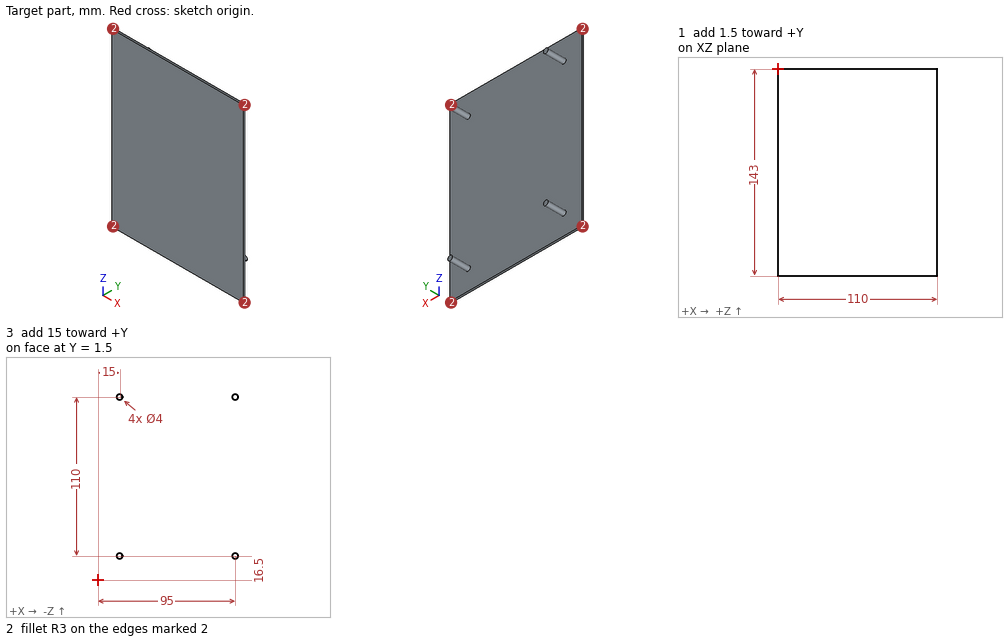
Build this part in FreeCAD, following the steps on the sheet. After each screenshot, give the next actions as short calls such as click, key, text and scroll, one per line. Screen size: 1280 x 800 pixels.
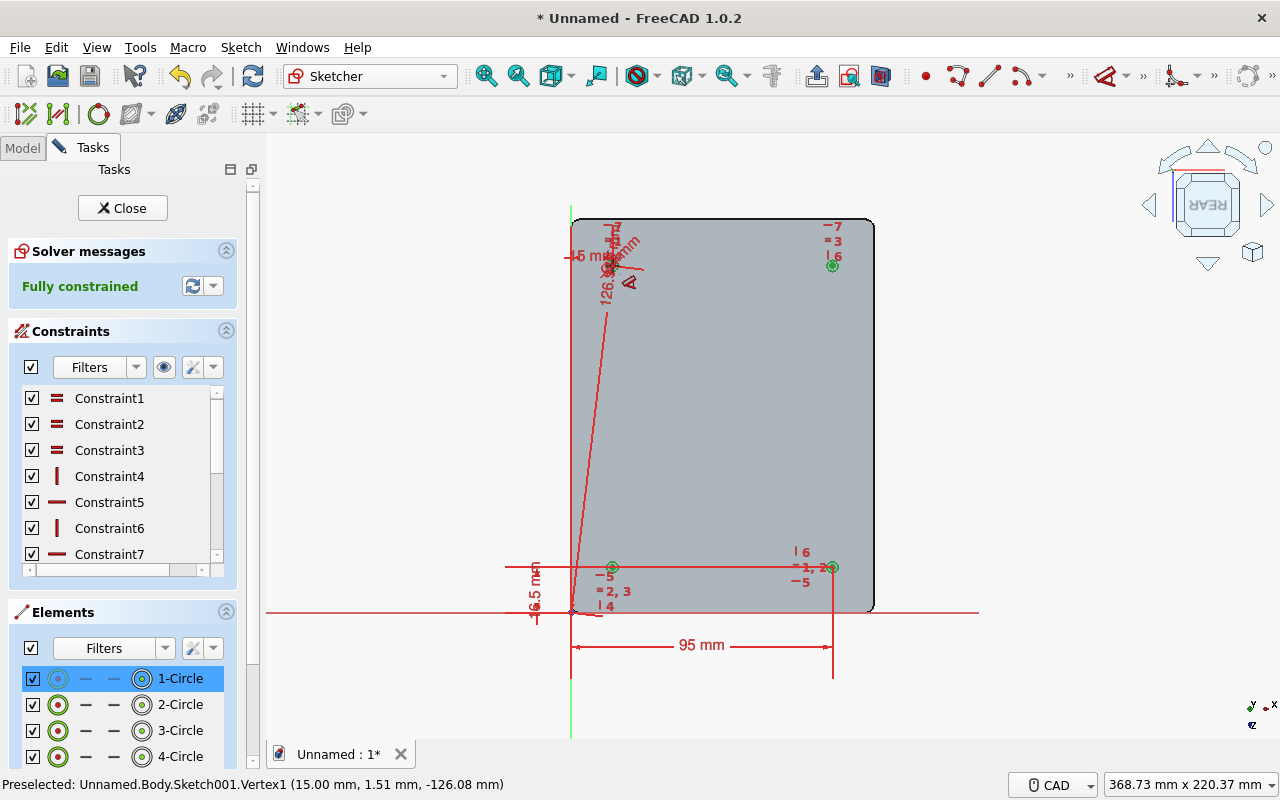
click(833, 567)
click(867, 417)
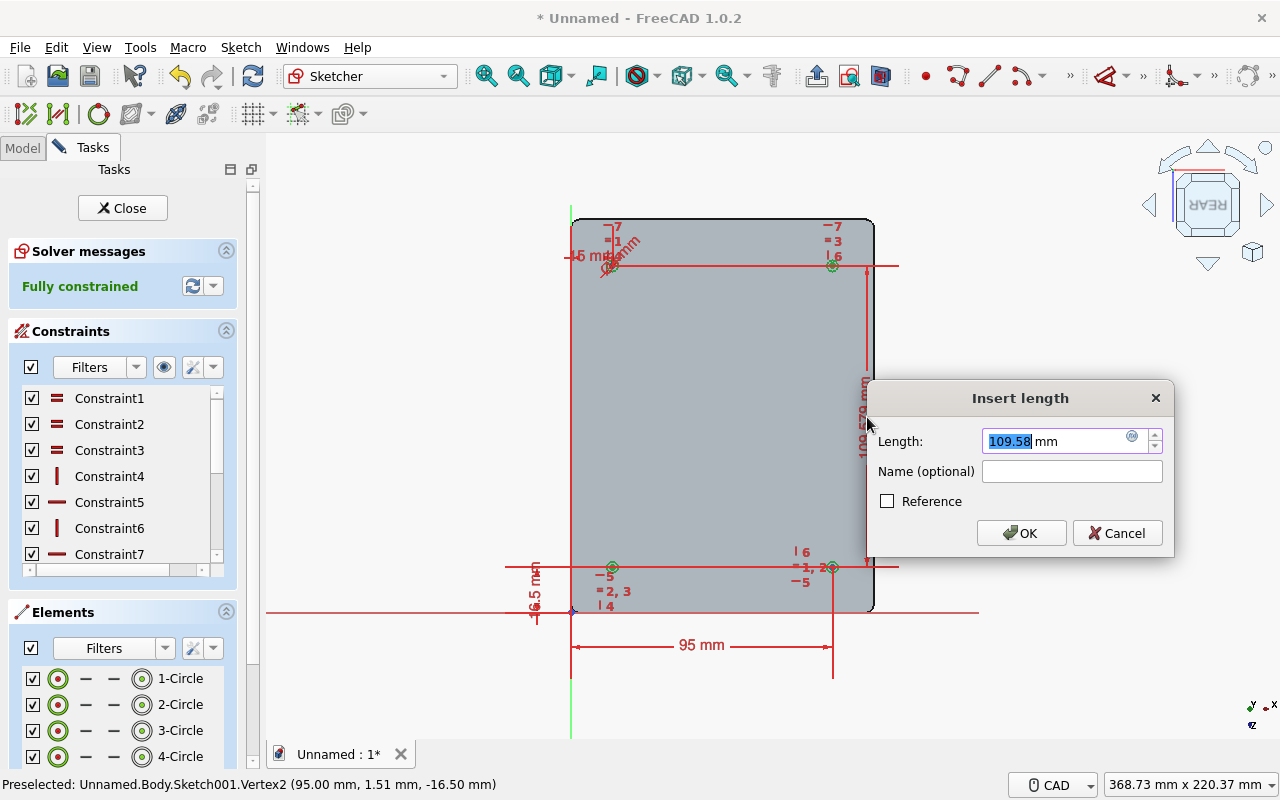
text(110)
key(Return)
key(Escape)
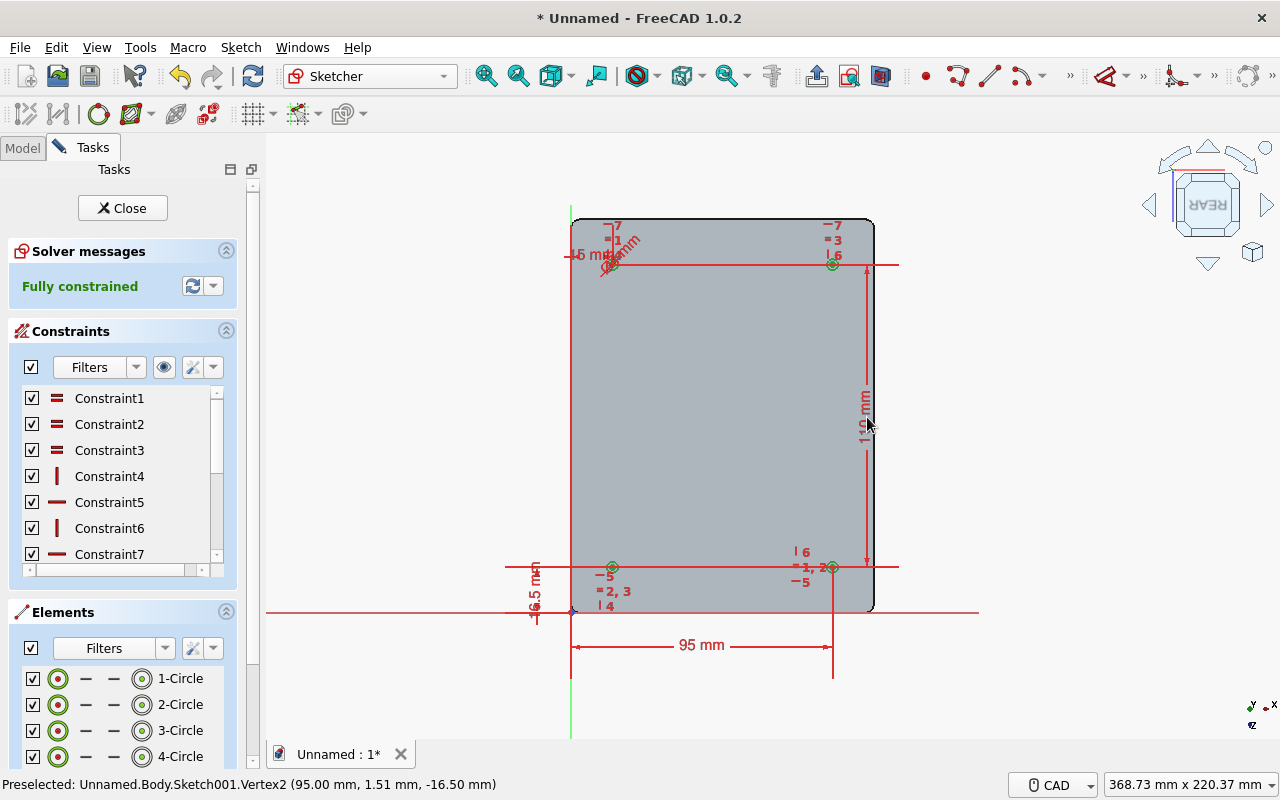
click(123, 208)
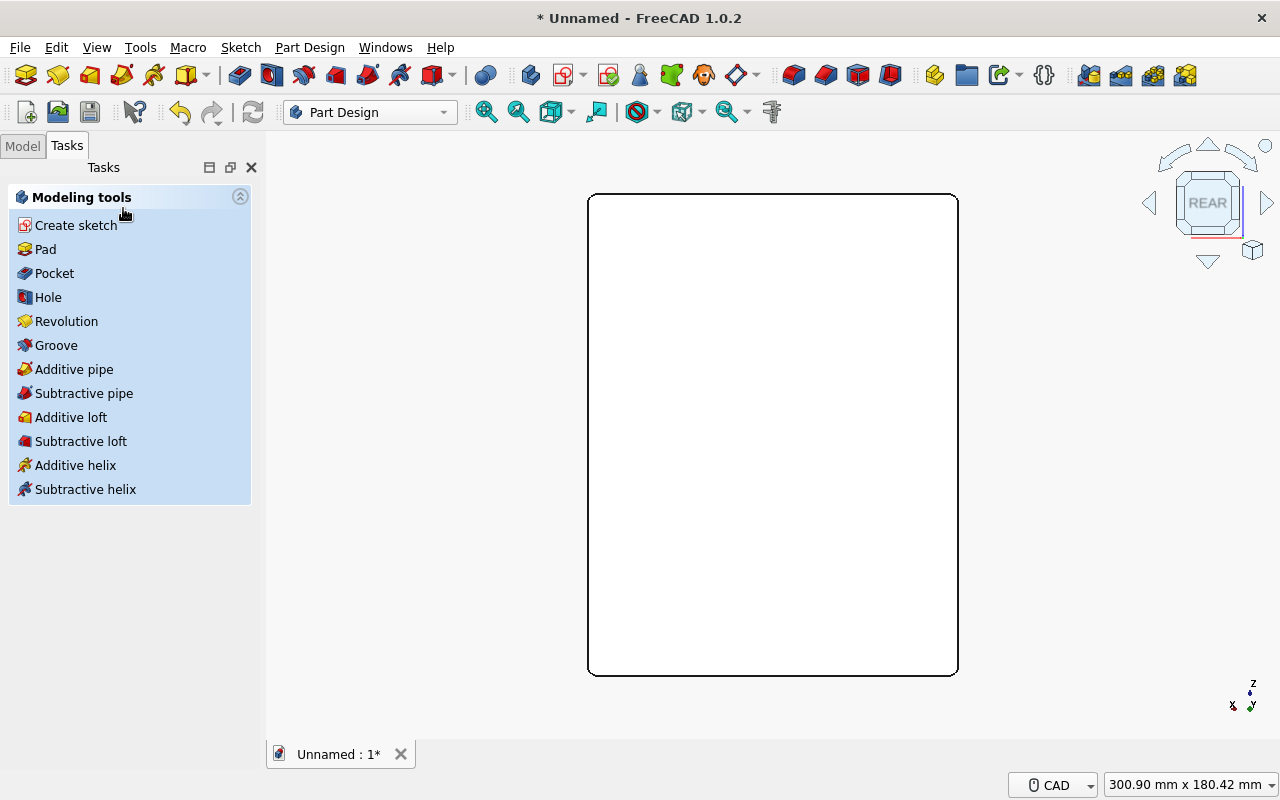
click(26, 76)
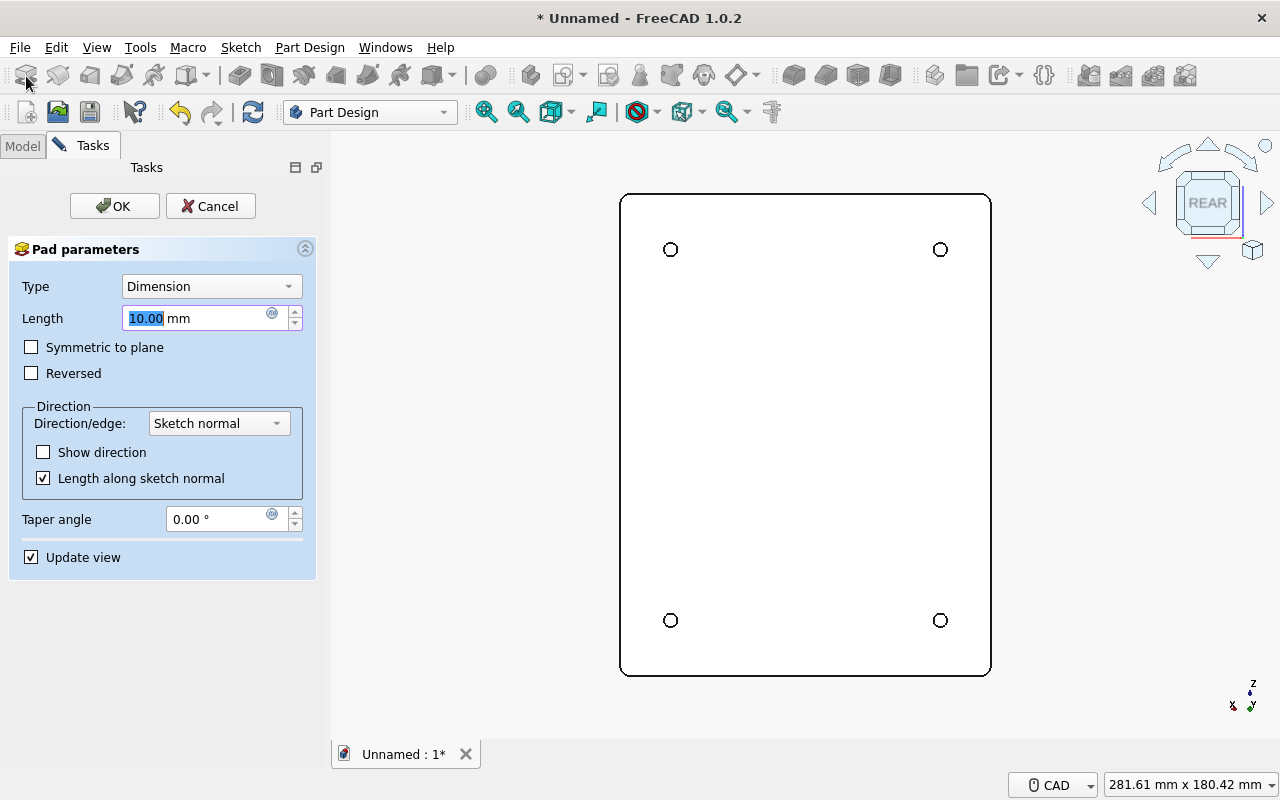
text(15)
key(Tab)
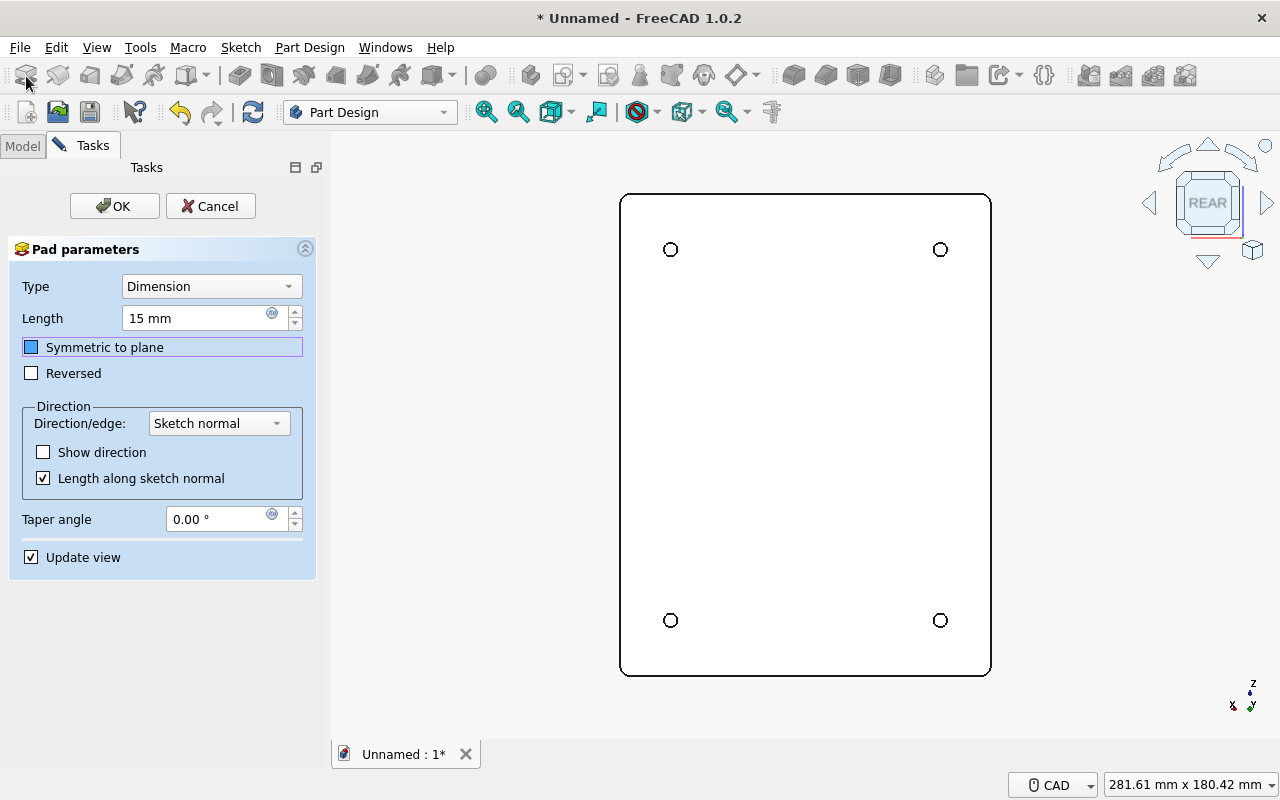
click(115, 206)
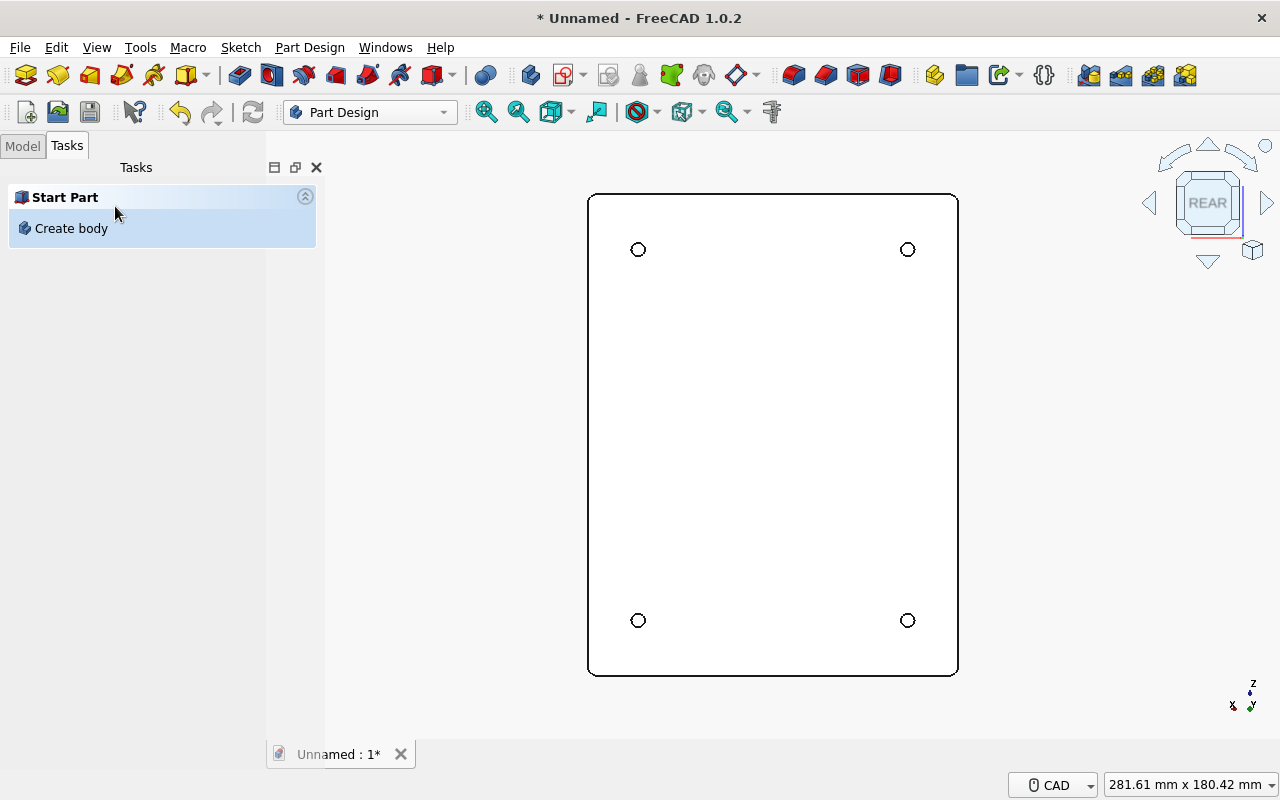
key(0)